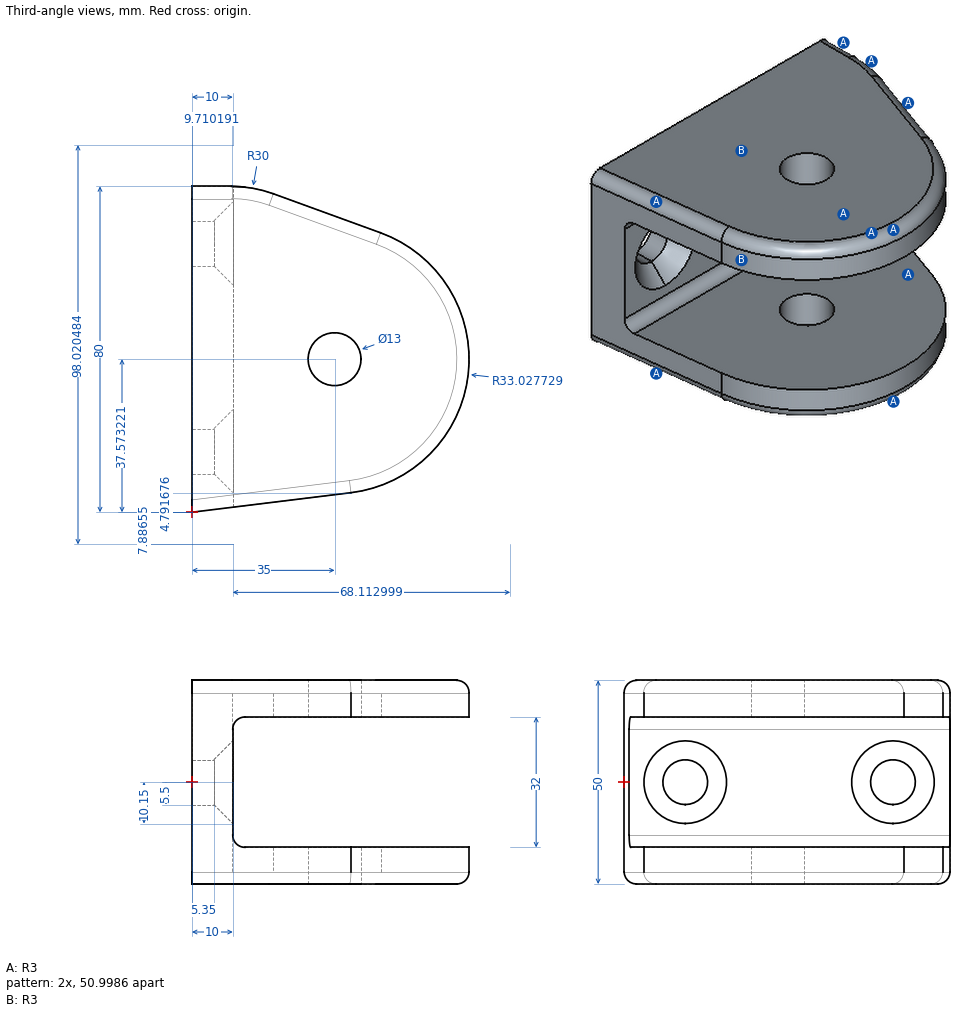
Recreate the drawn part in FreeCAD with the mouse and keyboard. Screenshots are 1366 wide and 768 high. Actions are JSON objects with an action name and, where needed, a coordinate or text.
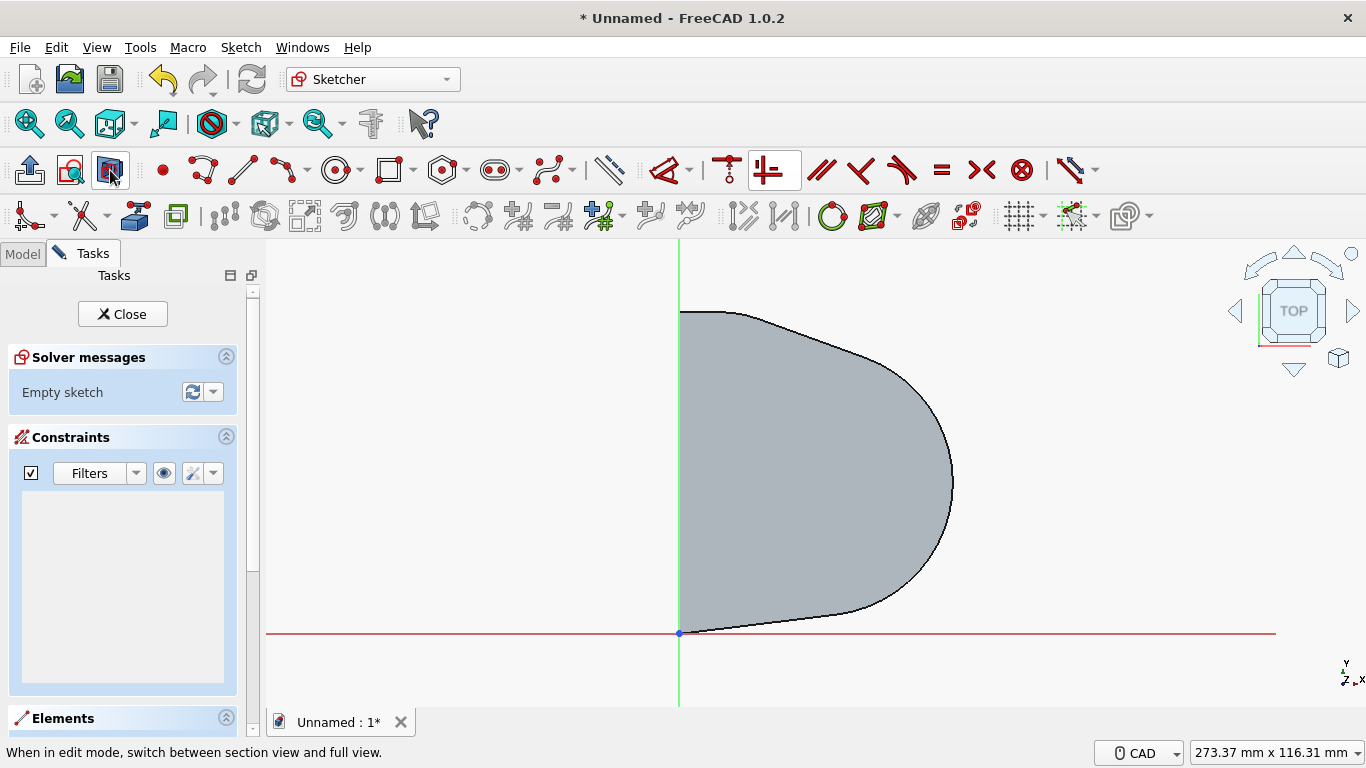
{"action": "scroll", "coordinate": [567, 482], "scroll_direction": "down", "scroll_amount": 2}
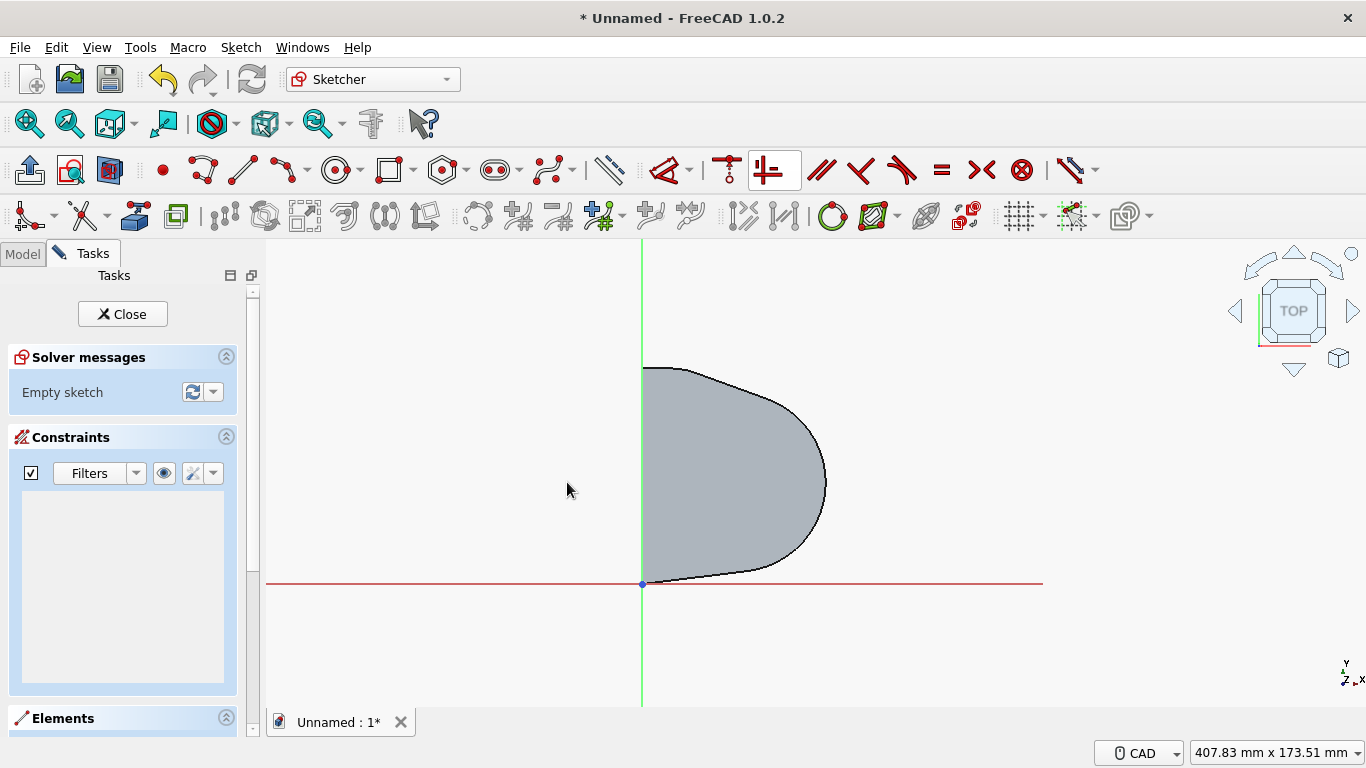
{"action": "left_click", "coordinate": [390, 170]}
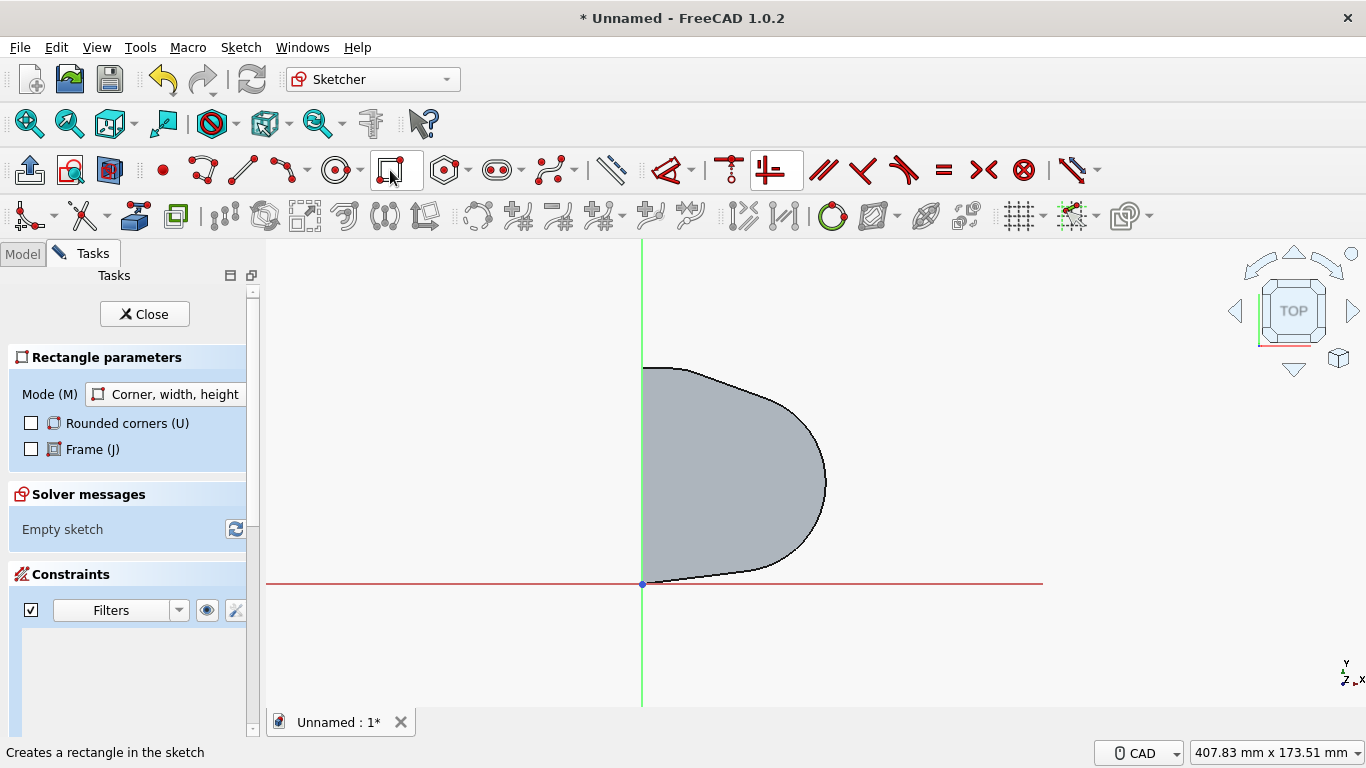
{"action": "left_click", "coordinate": [669, 341]}
{"action": "left_click", "coordinate": [853, 605]}
{"action": "key", "text": "Escape"}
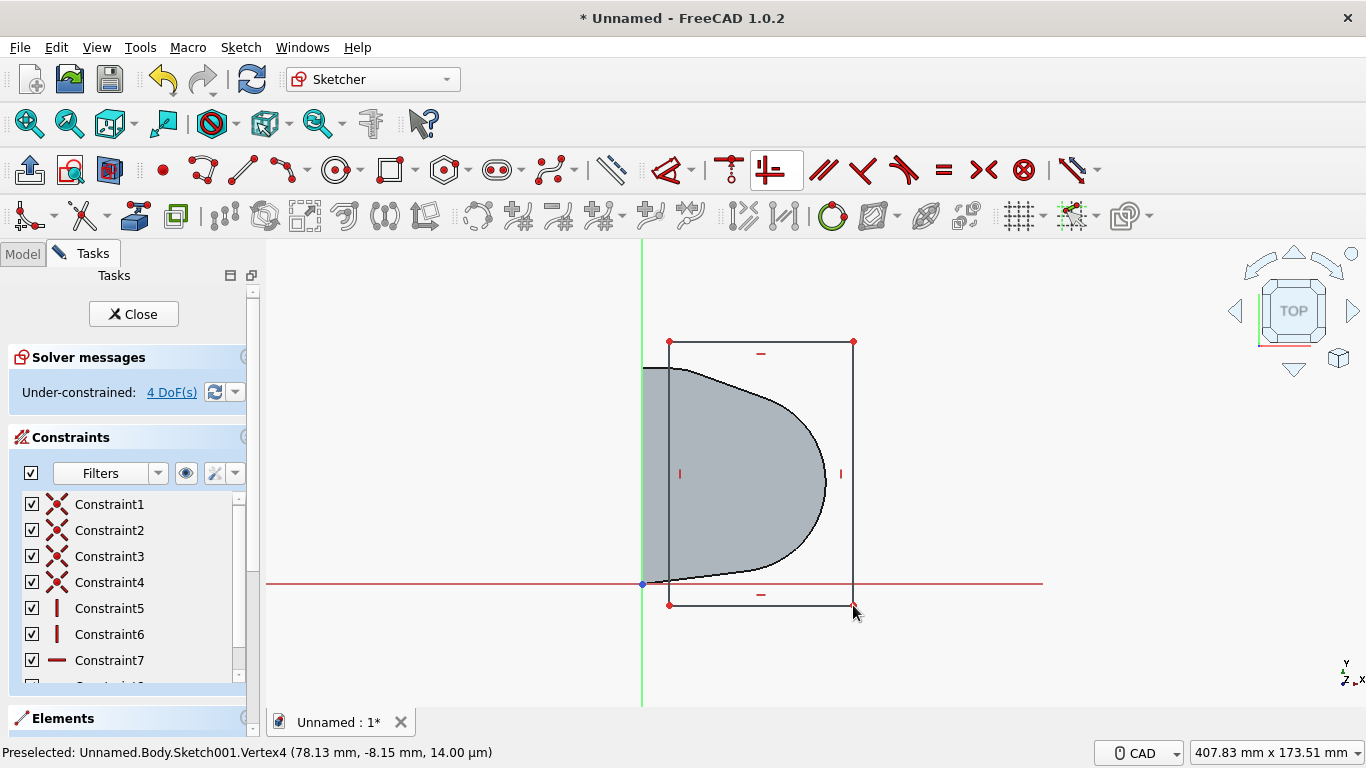
{"action": "left_click", "coordinate": [666, 170]}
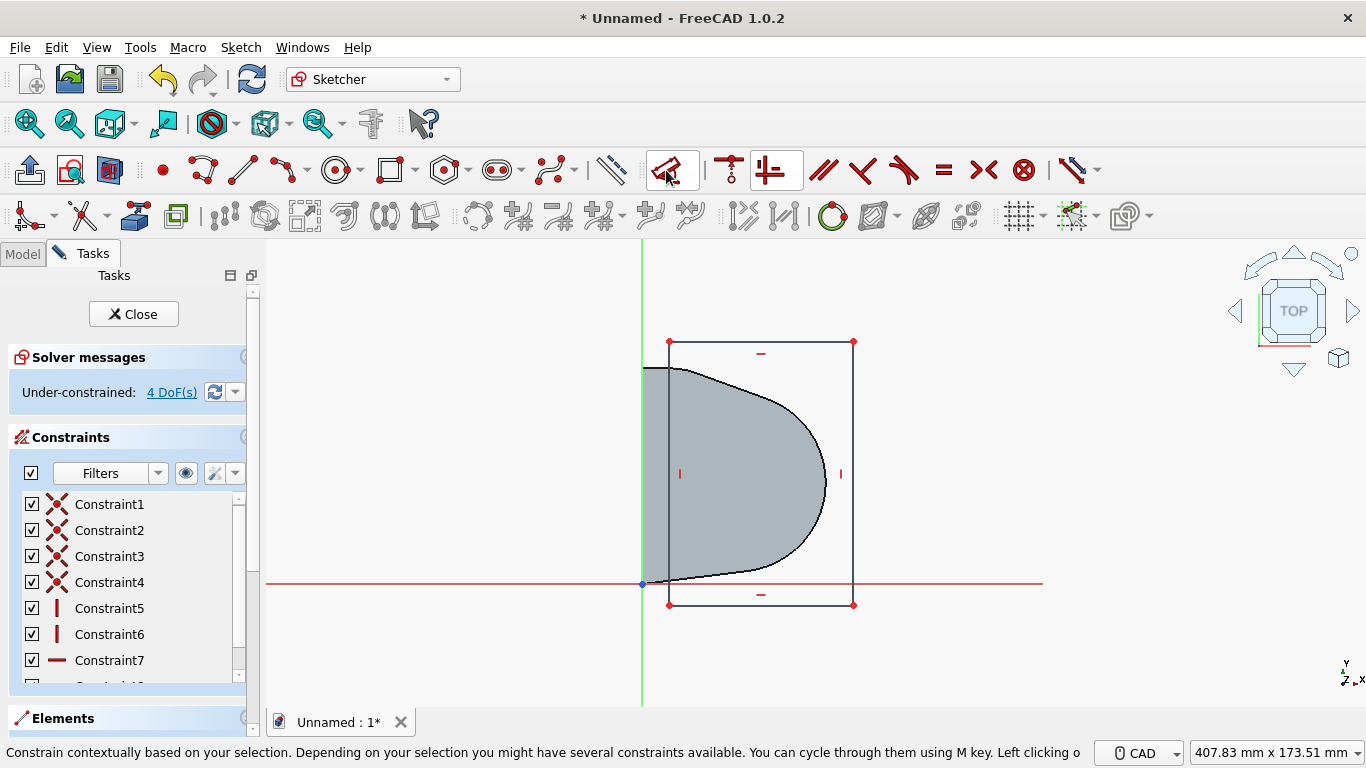
{"action": "scroll", "coordinate": [669, 342], "scroll_direction": "up", "scroll_amount": 2}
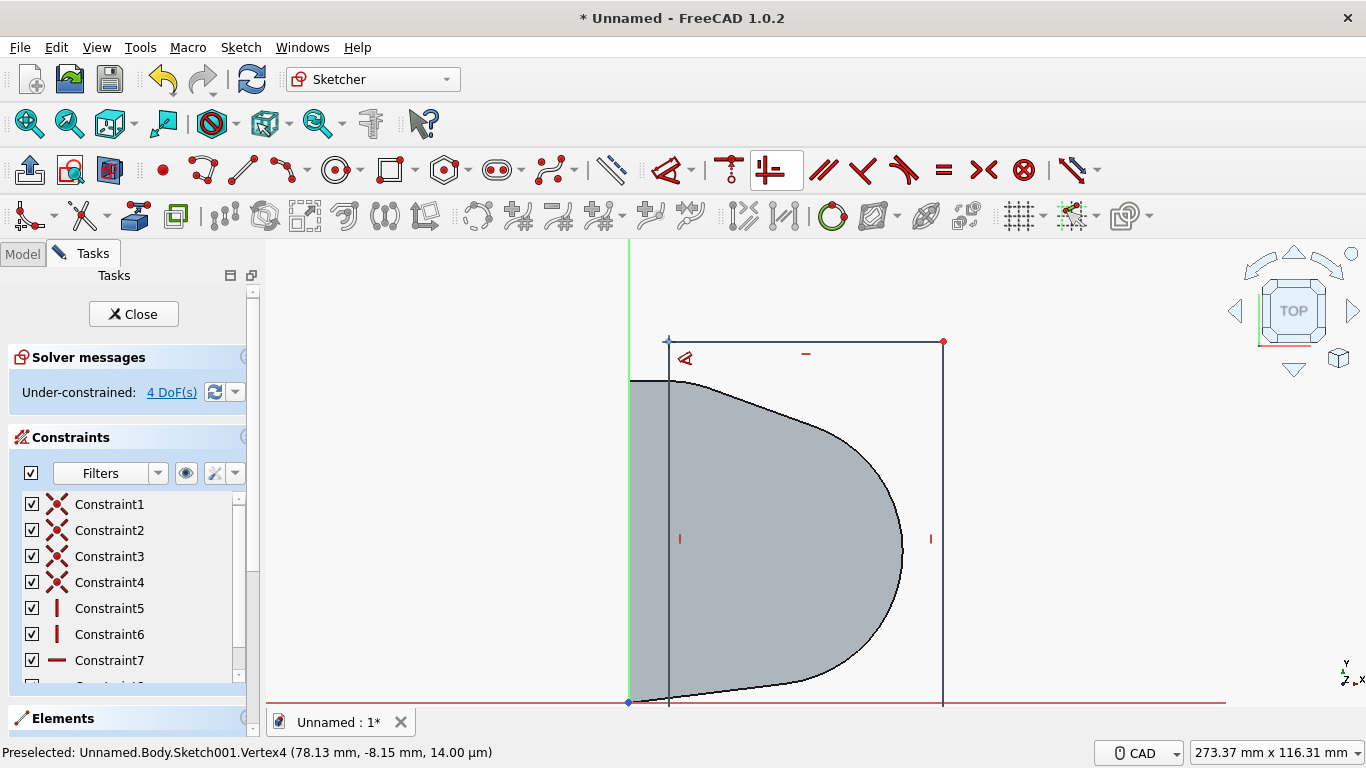
{"action": "left_click", "coordinate": [669, 342]}
{"action": "left_click", "coordinate": [649, 308]}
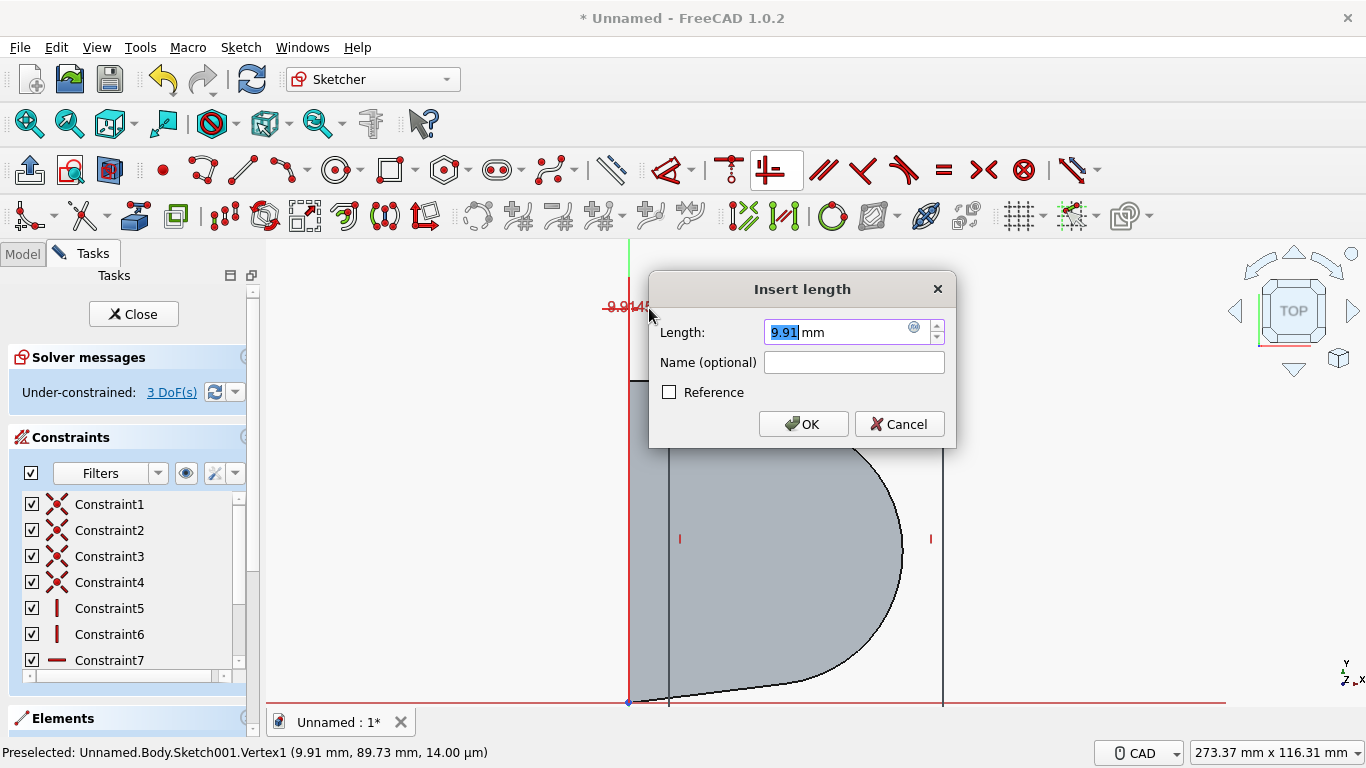
{"action": "type", "text": "10"}
{"action": "key", "text": "Return"}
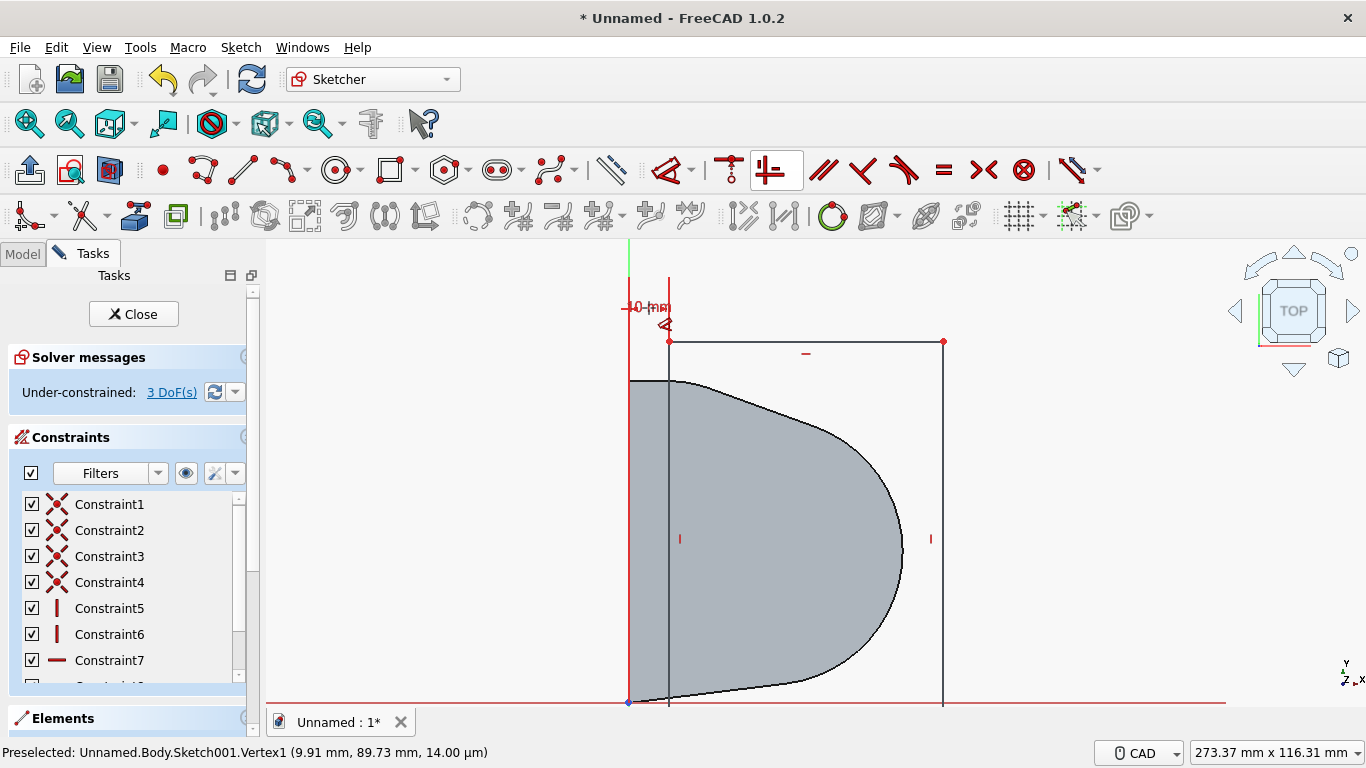
{"action": "scroll", "coordinate": [669, 342], "scroll_direction": "down", "scroll_amount": 2}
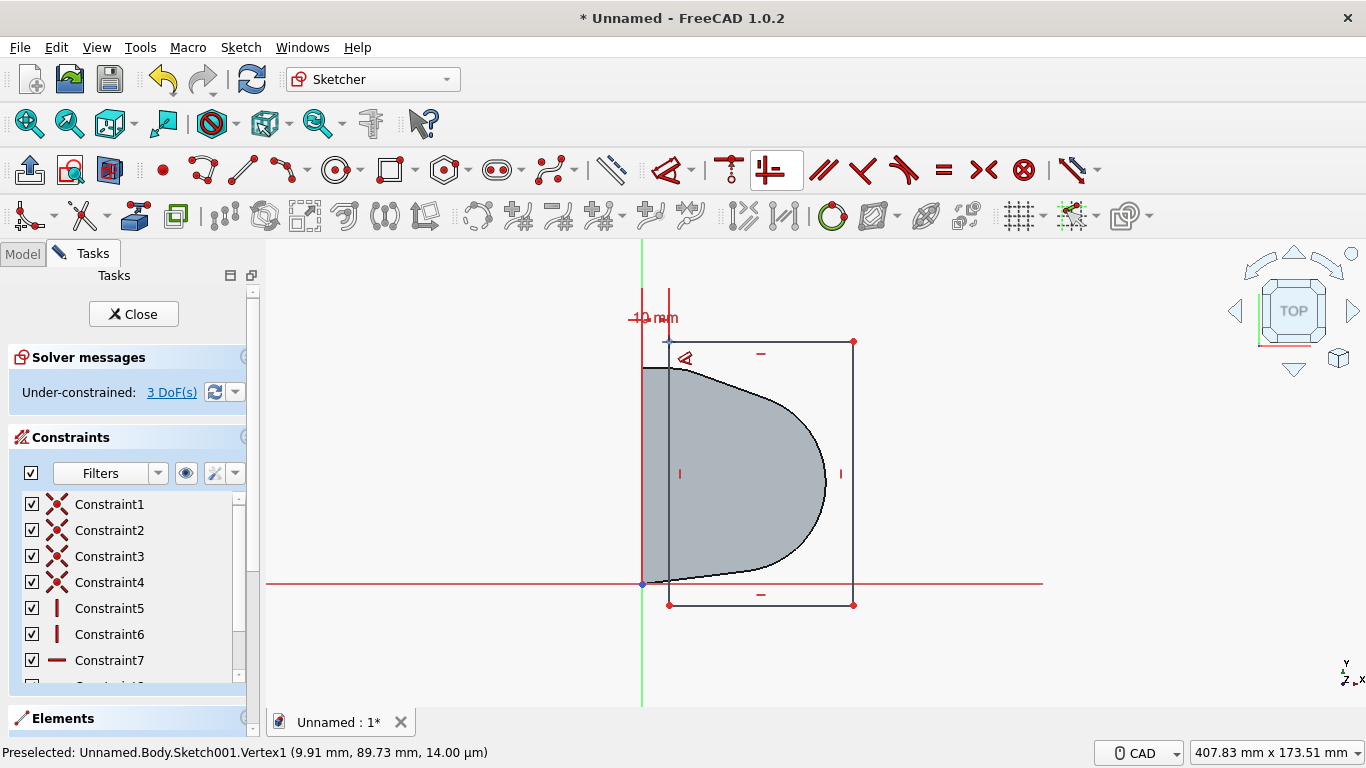
{"action": "scroll", "coordinate": [669, 606], "scroll_direction": "up", "scroll_amount": 4}